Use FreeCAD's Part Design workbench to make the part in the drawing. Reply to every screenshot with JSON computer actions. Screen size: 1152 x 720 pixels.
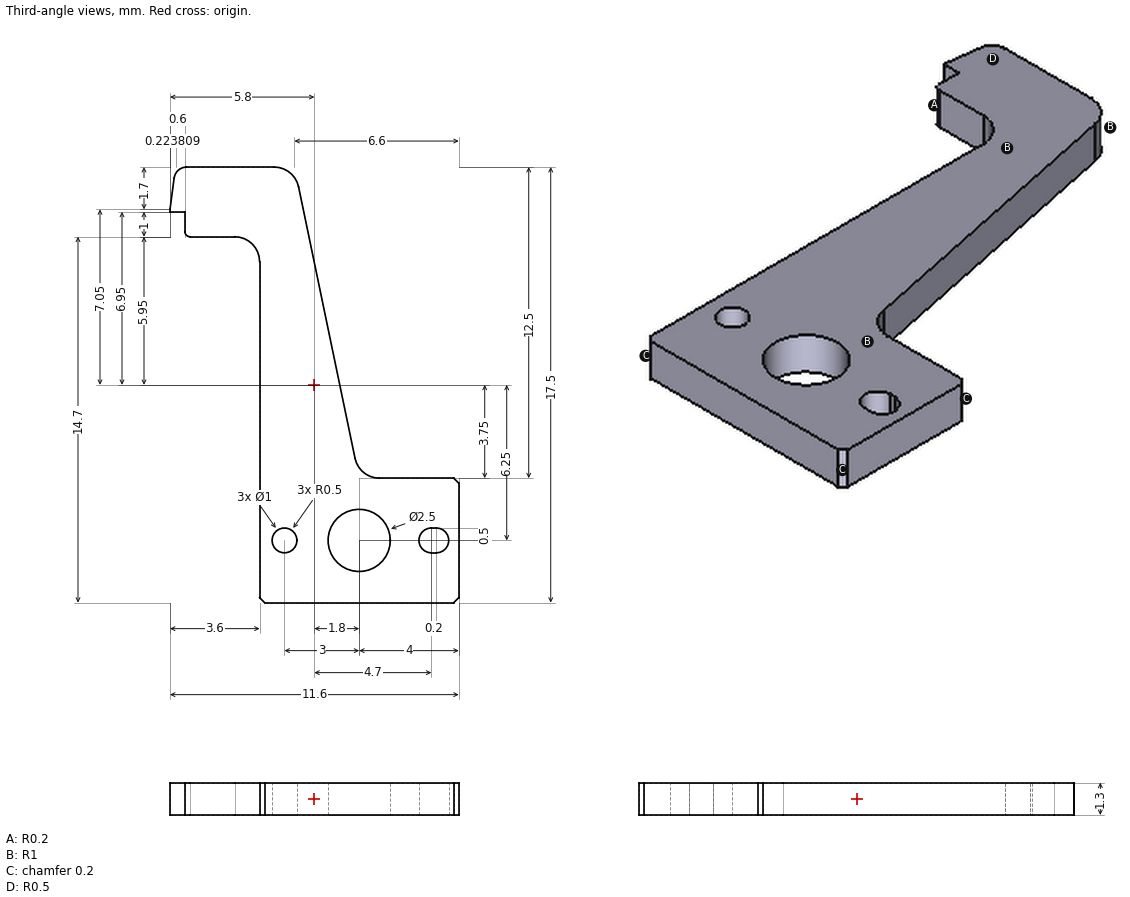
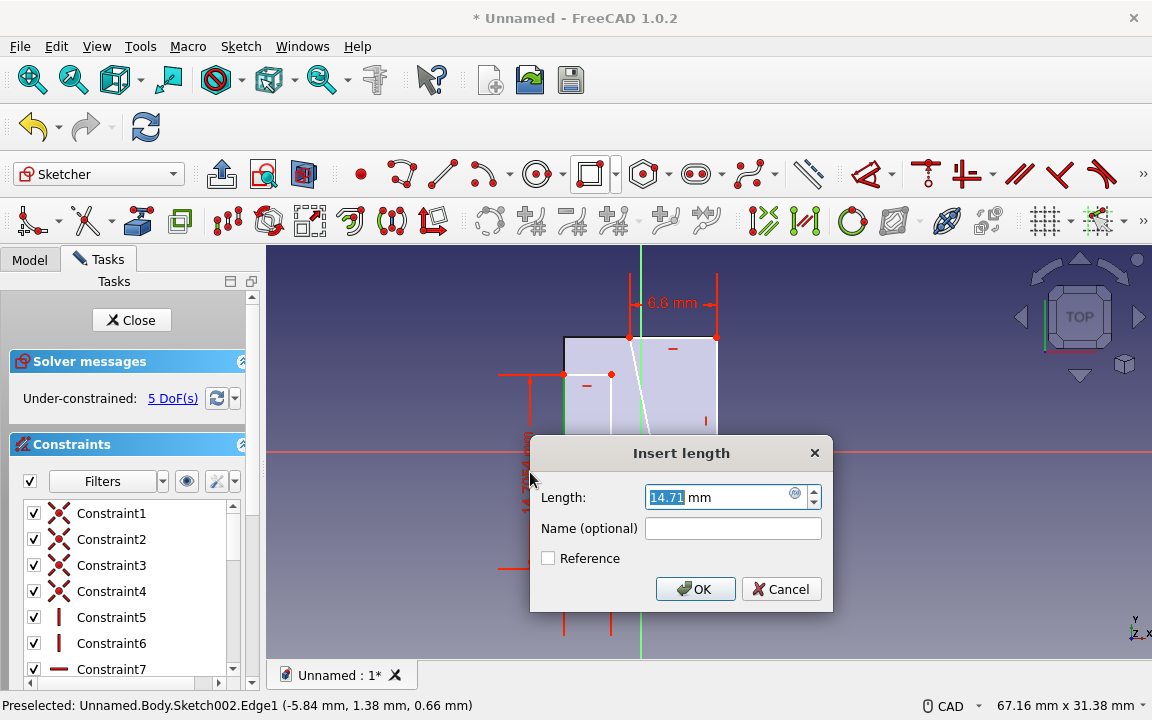
{"action": "type", "text": "14.7"}
{"action": "key", "text": "Return"}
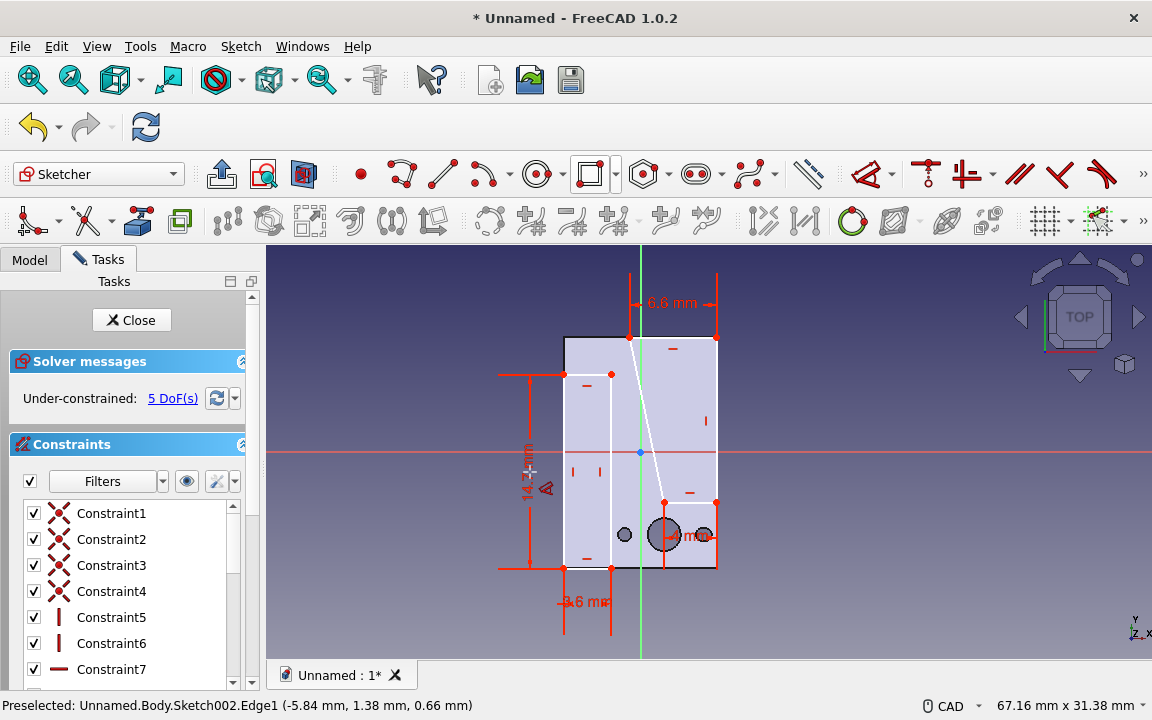
{"action": "left_click", "coordinate": [717, 453]}
{"action": "left_click", "coordinate": [751, 420]}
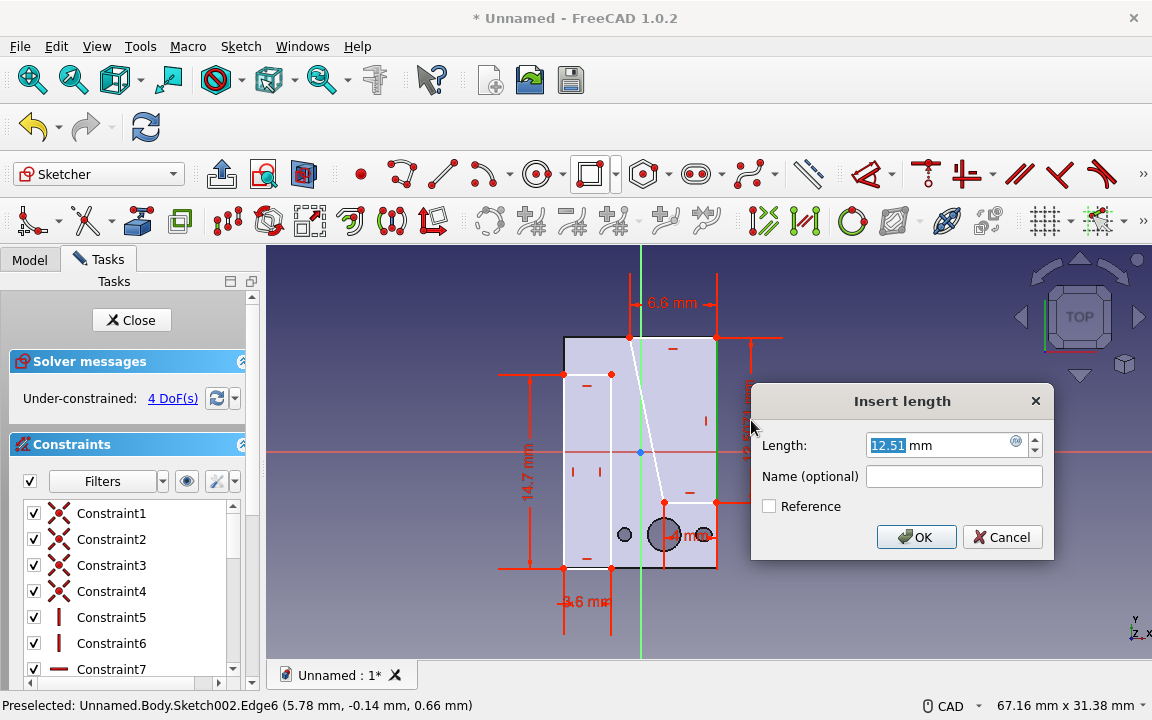
{"action": "type", "text": "12.5"}
{"action": "key", "text": "Return"}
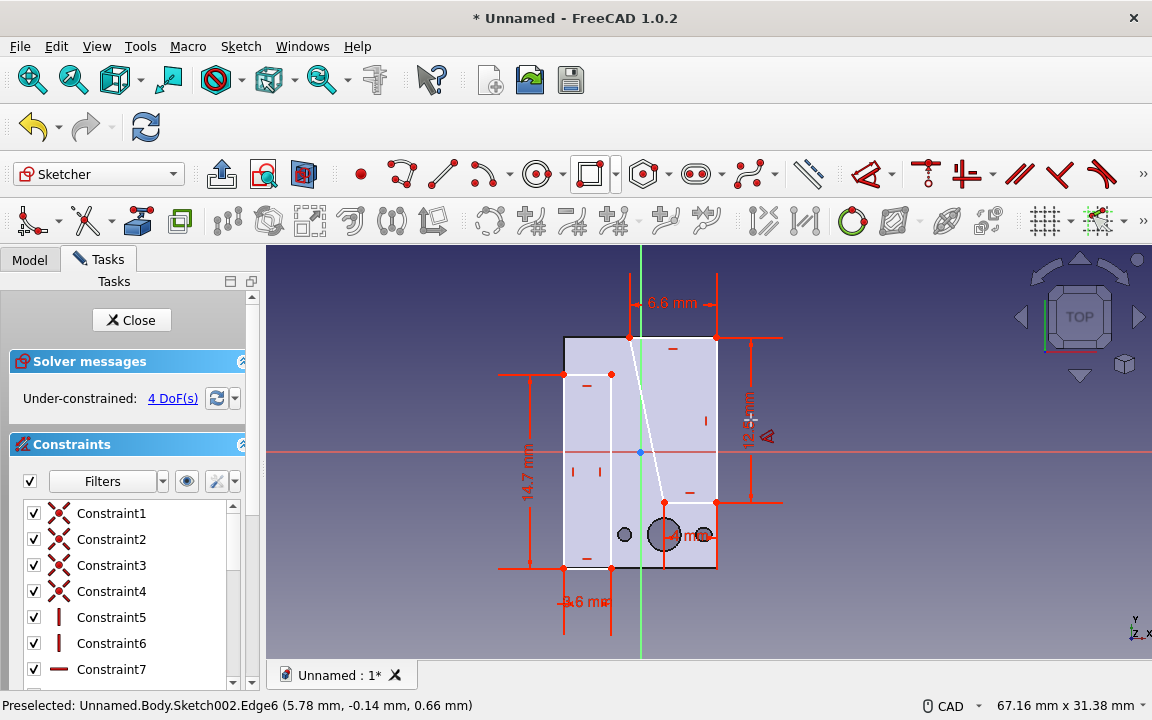
{"action": "left_click", "coordinate": [564, 375]}
{"action": "left_click", "coordinate": [602, 341]}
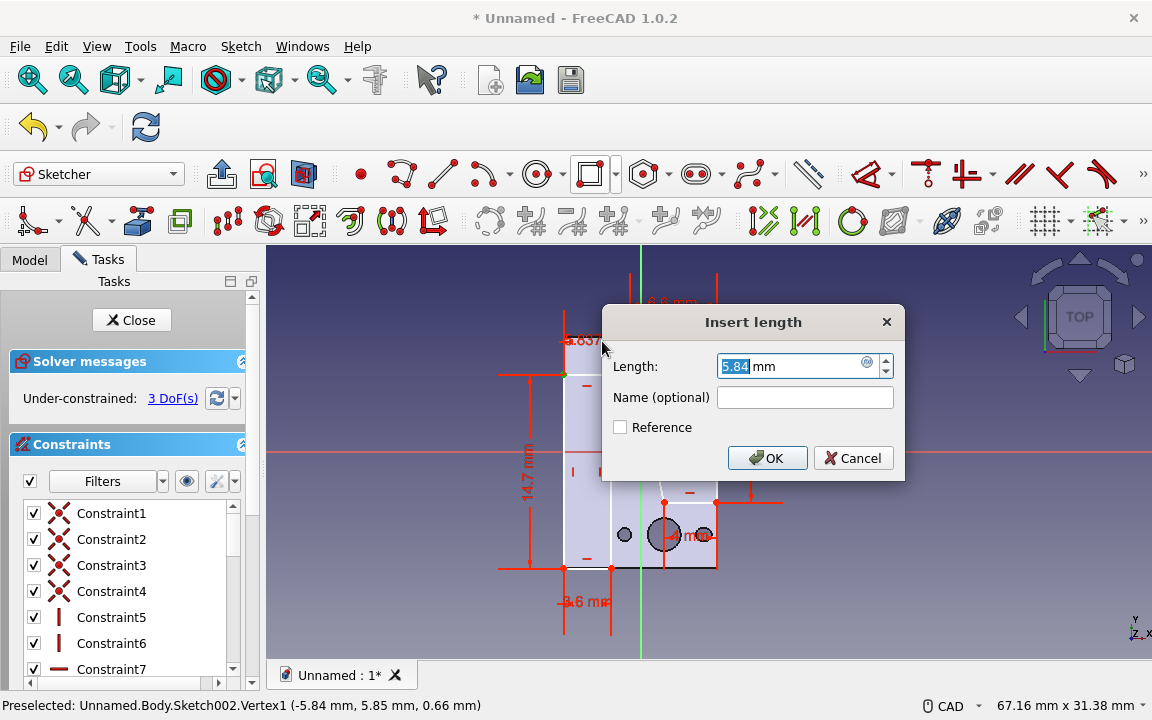
{"action": "type", "text": "5.8"}
{"action": "key", "text": "Return"}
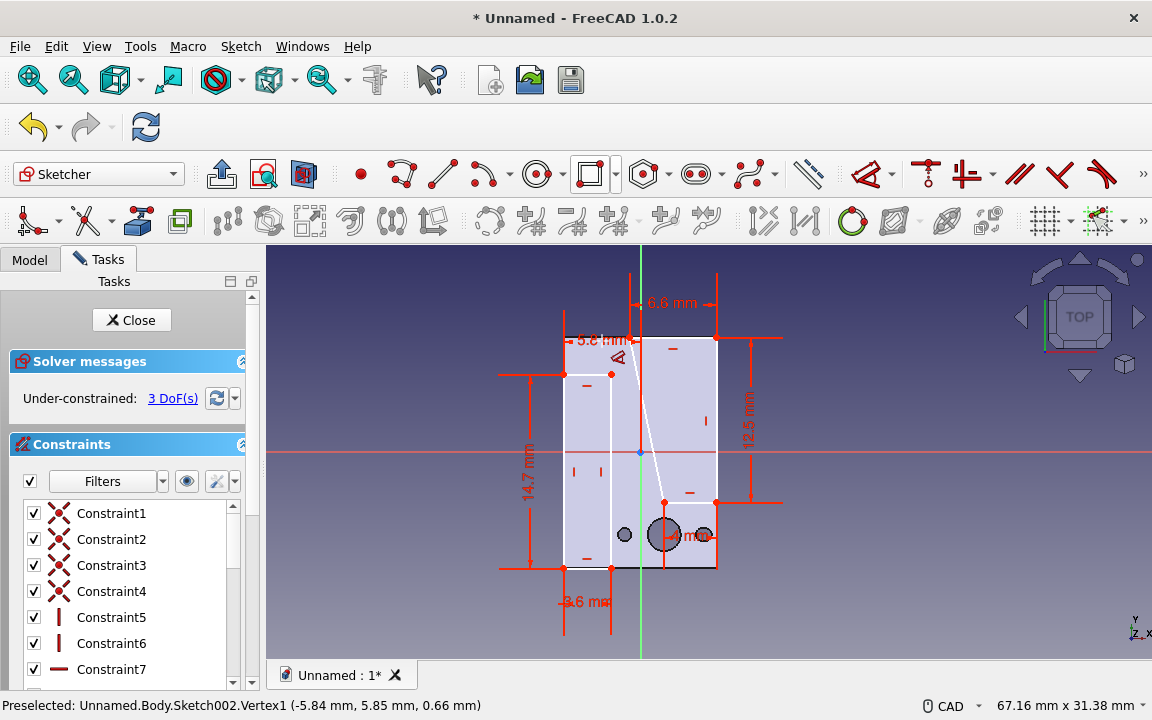
{"action": "scroll", "coordinate": [664, 503], "scroll_direction": "up", "scroll_amount": 3}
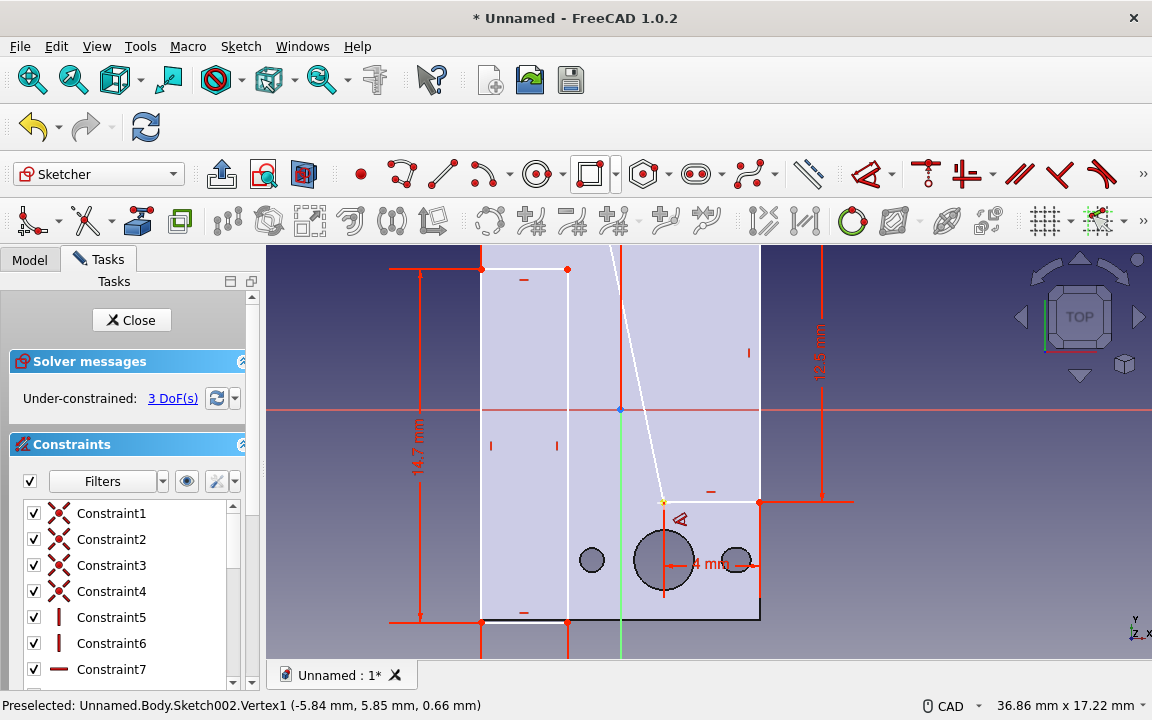
{"action": "left_click", "coordinate": [664, 502]}
{"action": "left_click", "coordinate": [642, 536]}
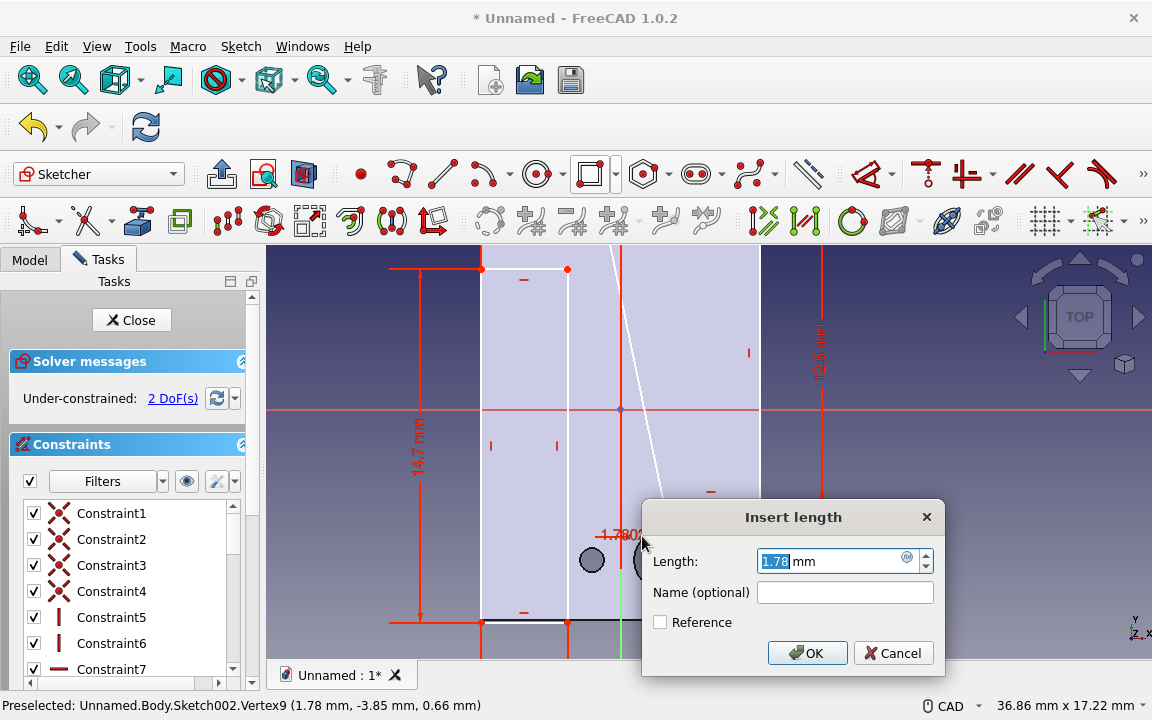
{"action": "type", "text": "1.8"}
{"action": "key", "text": "Return"}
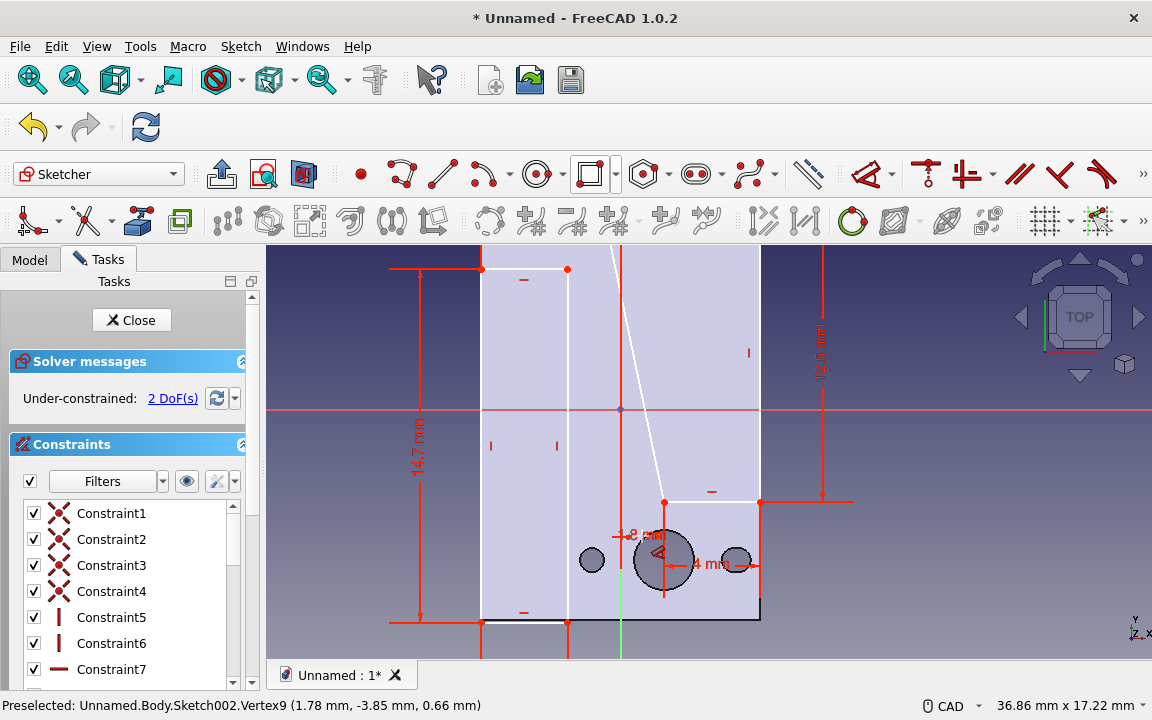
{"action": "scroll", "coordinate": [664, 503], "scroll_direction": "down", "scroll_amount": 3}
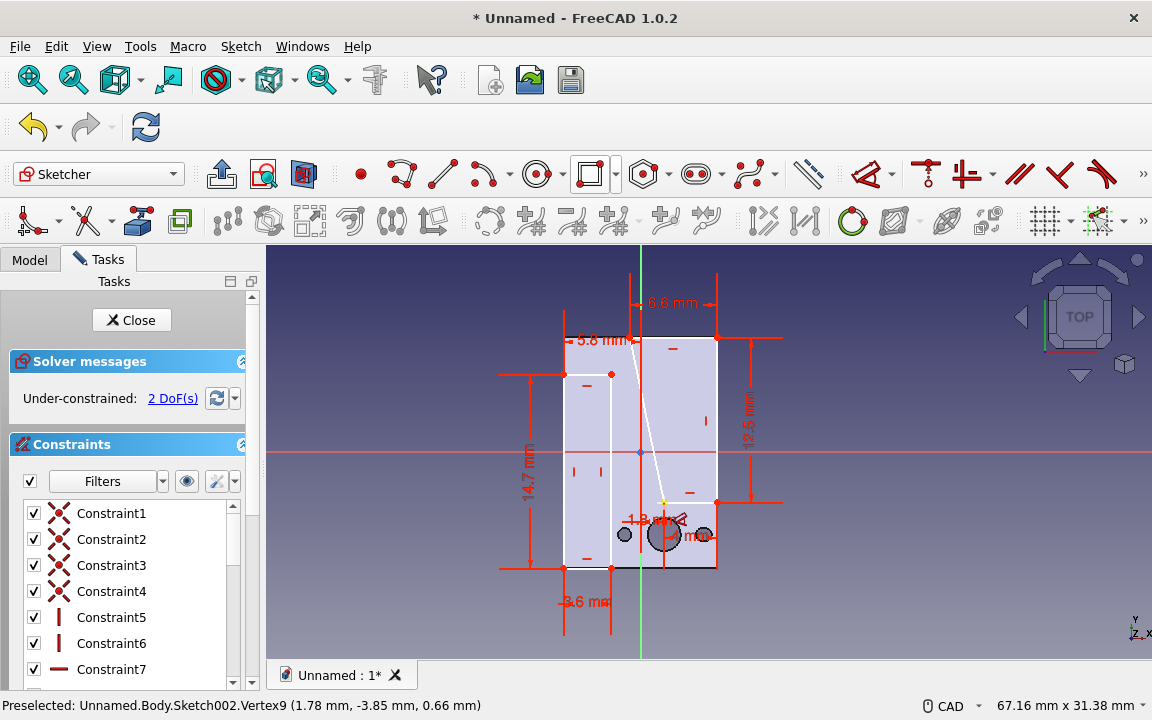
{"action": "left_click", "coordinate": [564, 375]}
{"action": "left_click", "coordinate": [530, 414]}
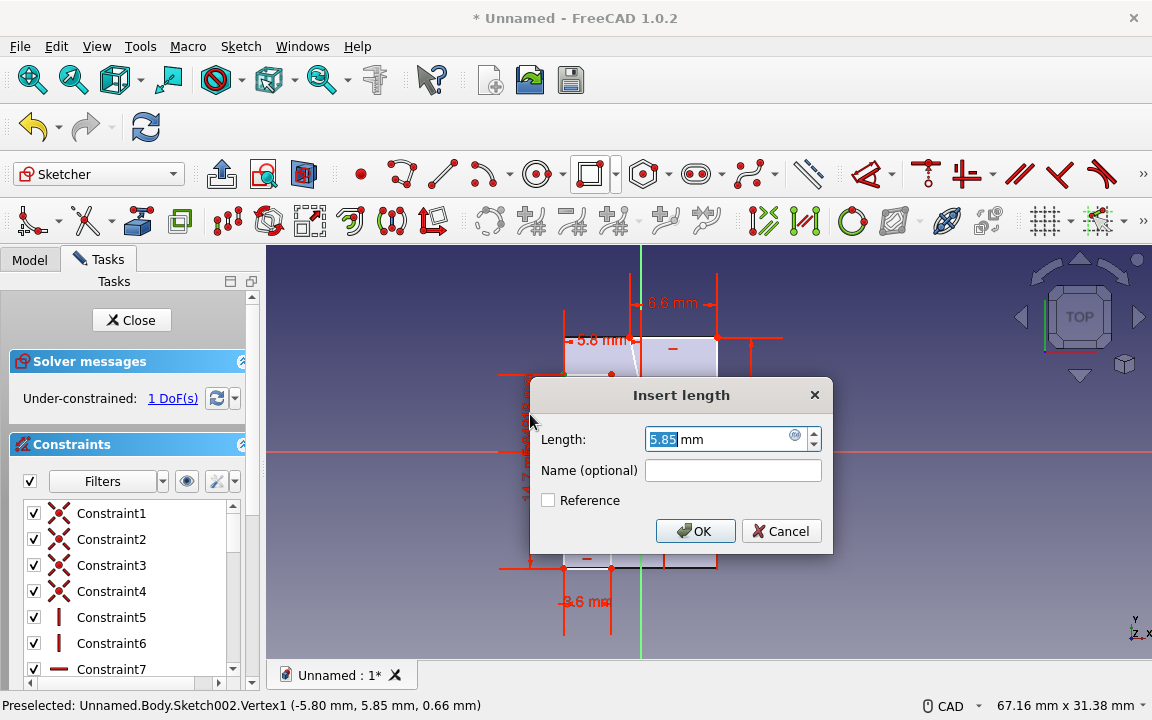
{"action": "type", "text": "5.95"}
{"action": "key", "text": "Return"}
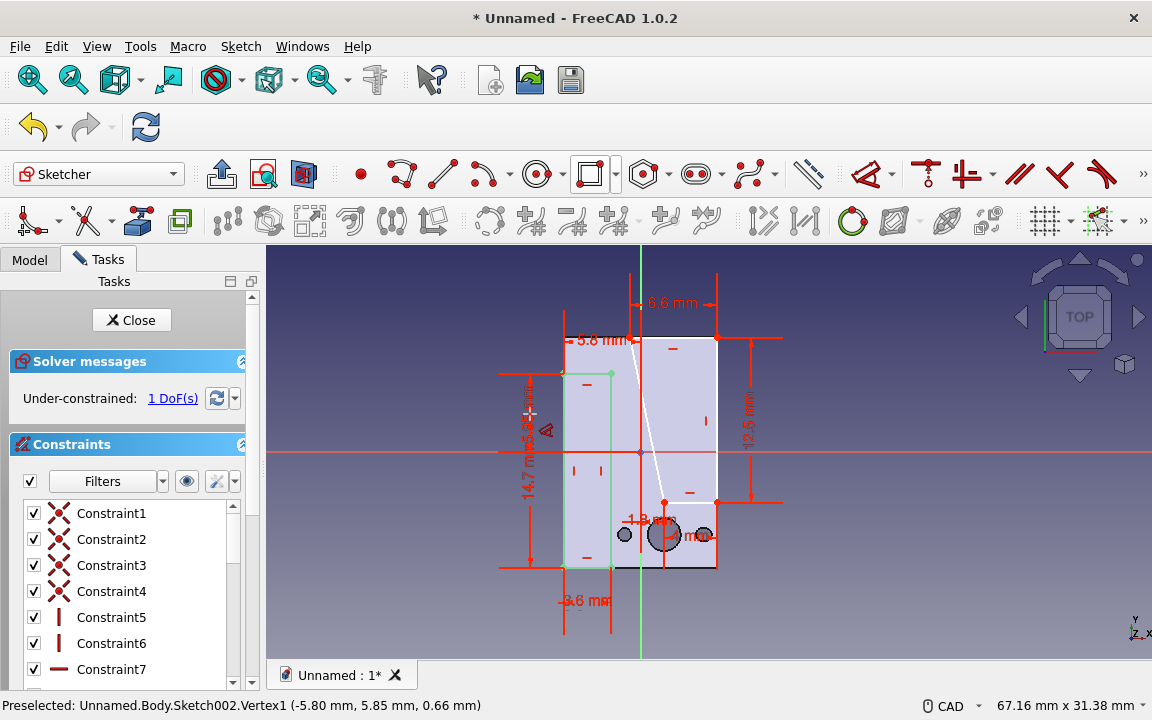
{"action": "left_click", "coordinate": [664, 503]}
{"action": "left_click", "coordinate": [698, 478]}